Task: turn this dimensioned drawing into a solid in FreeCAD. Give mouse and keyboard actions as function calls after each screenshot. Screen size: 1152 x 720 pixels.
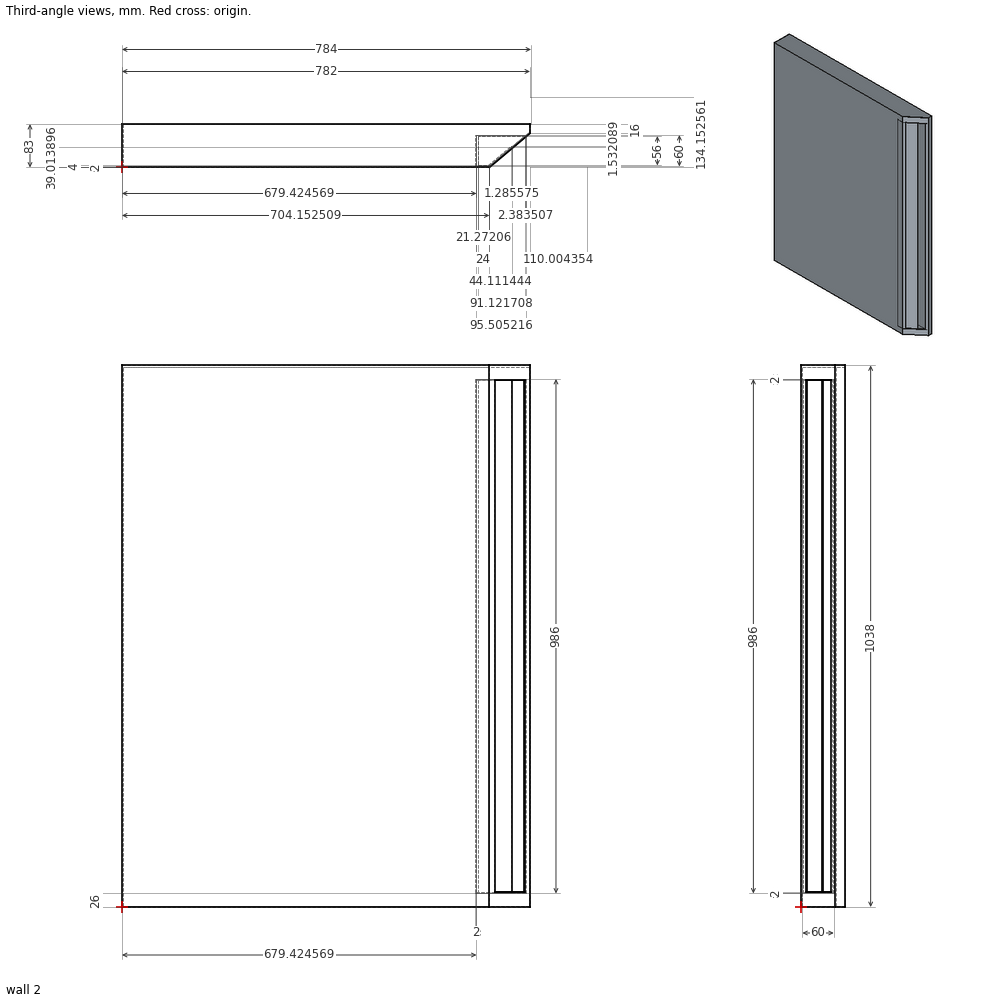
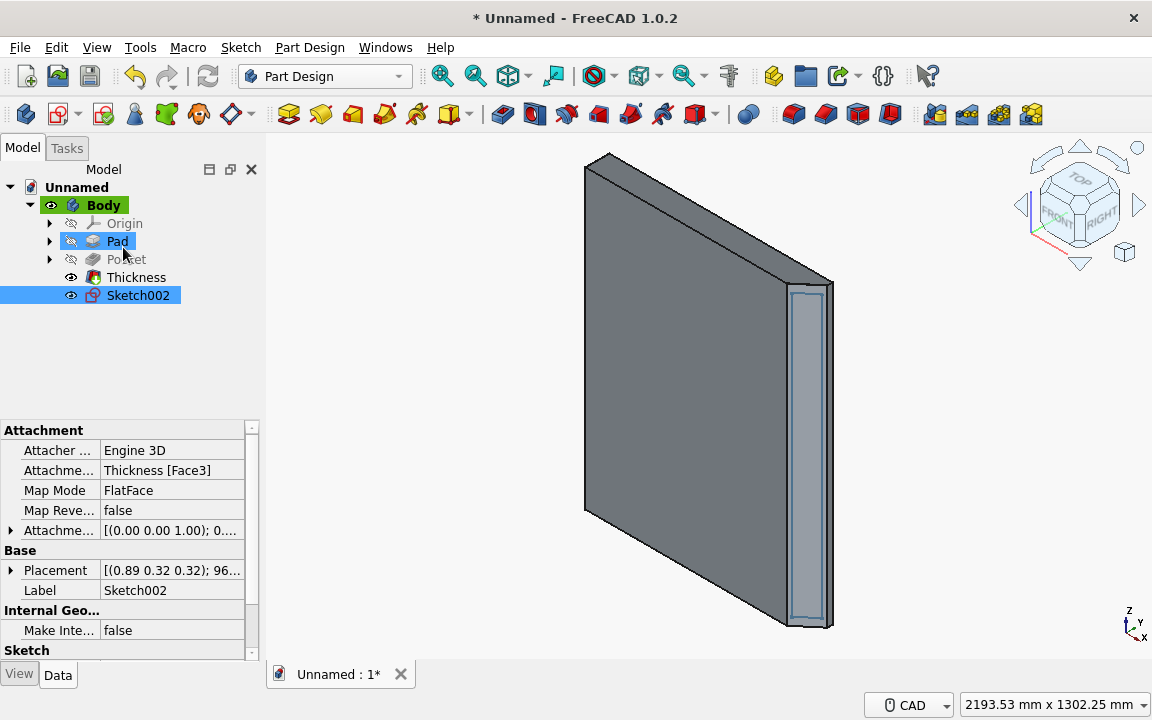
click(504, 114)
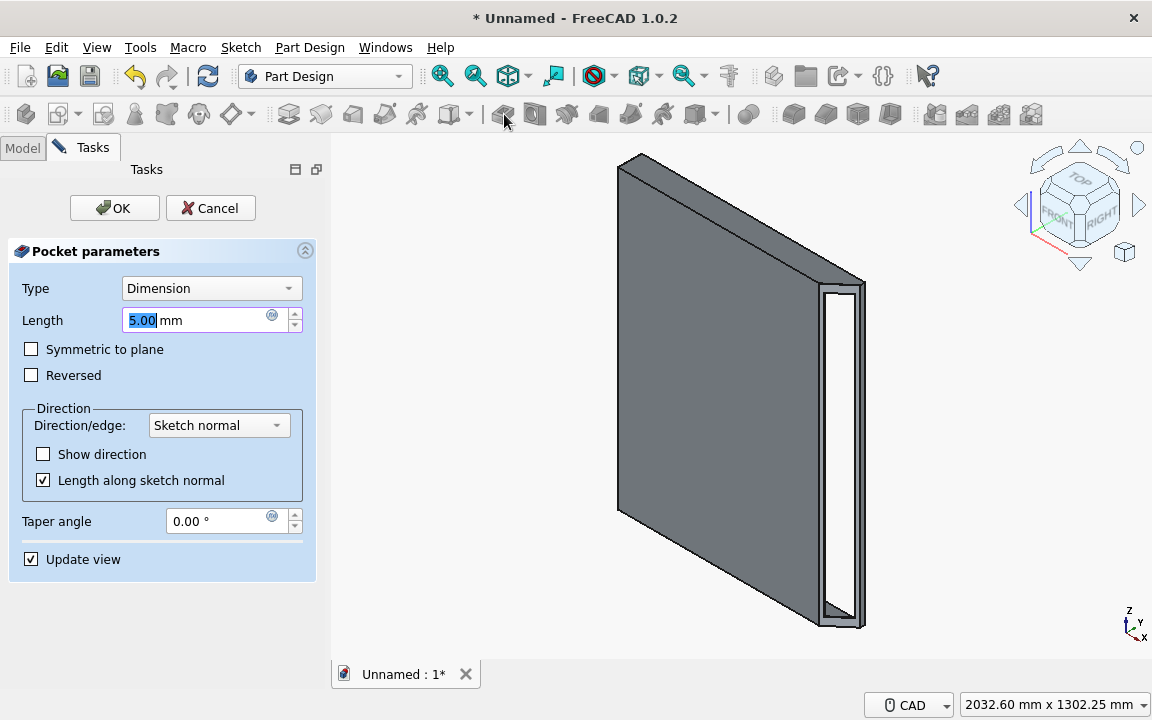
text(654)
key(Tab)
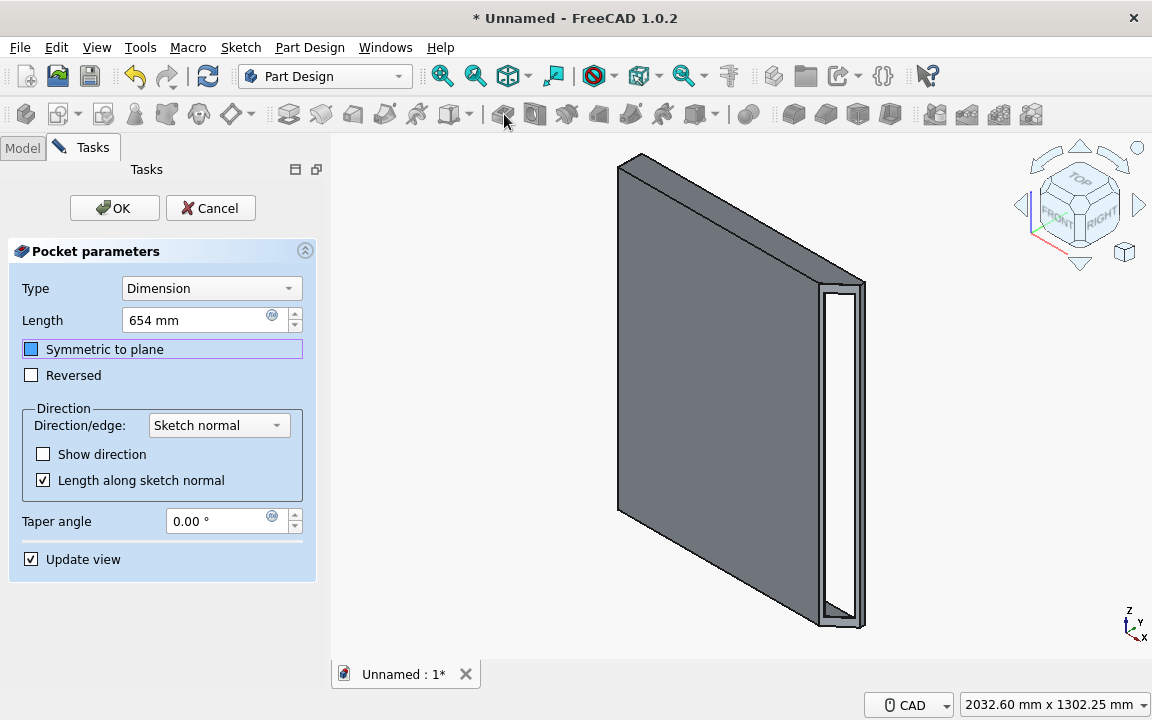
click(115, 208)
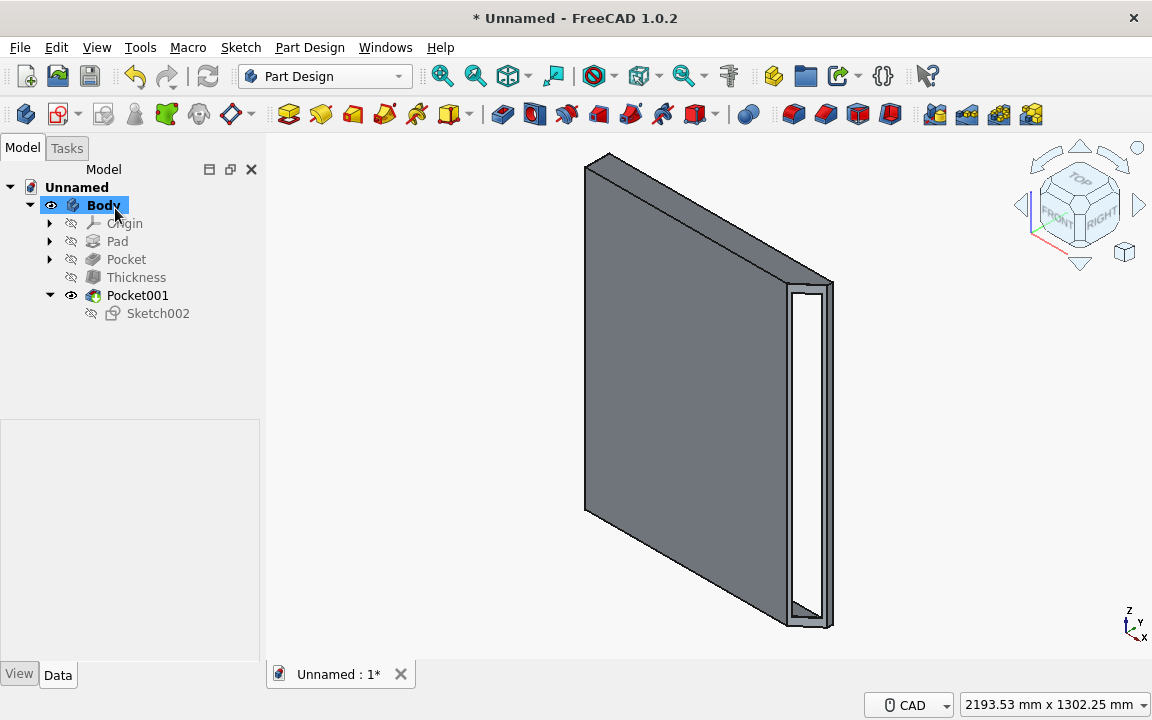
key(4)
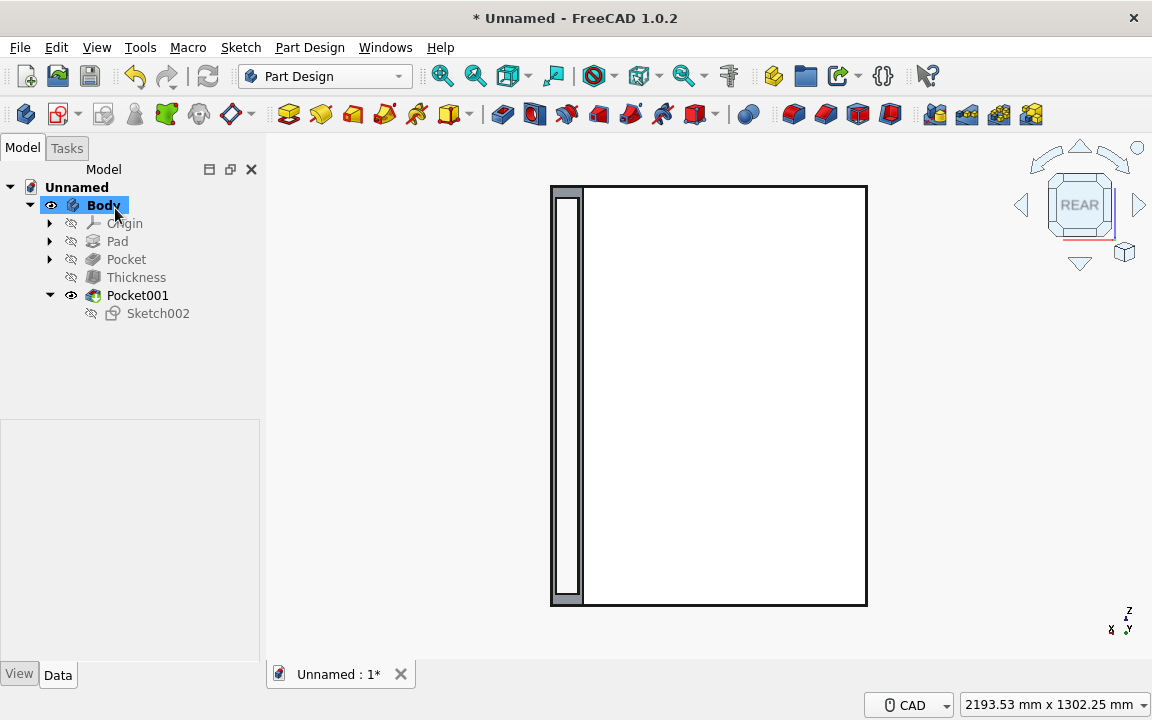
click(724, 335)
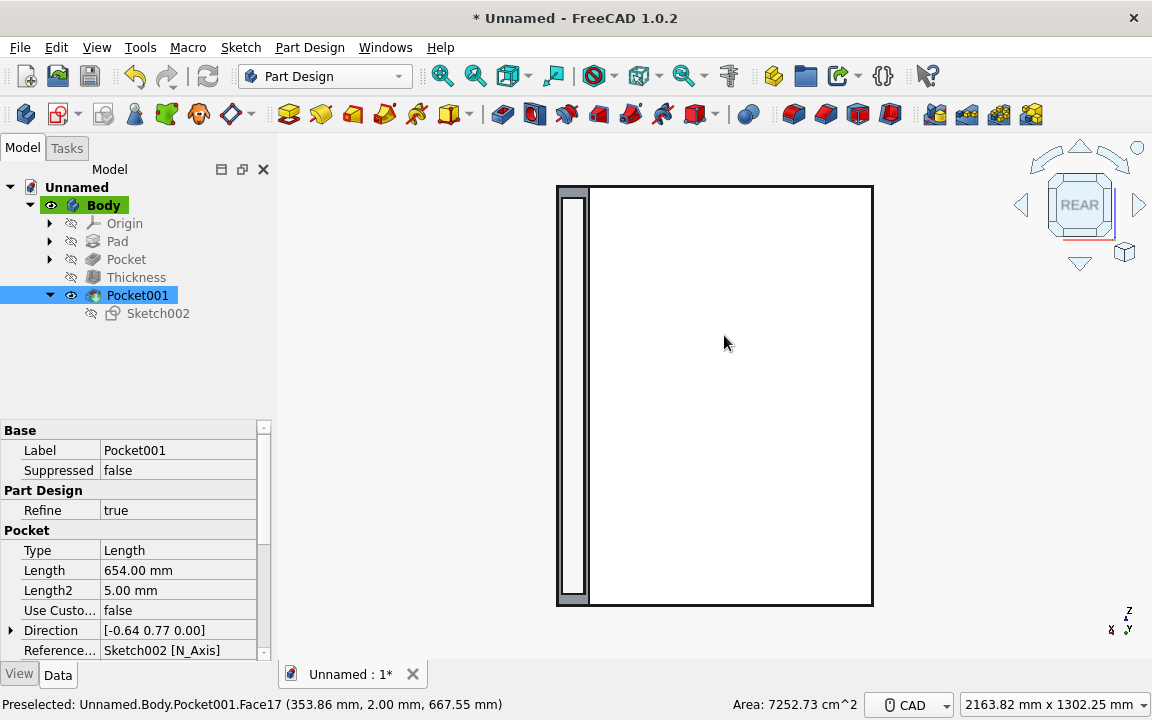
click(58, 114)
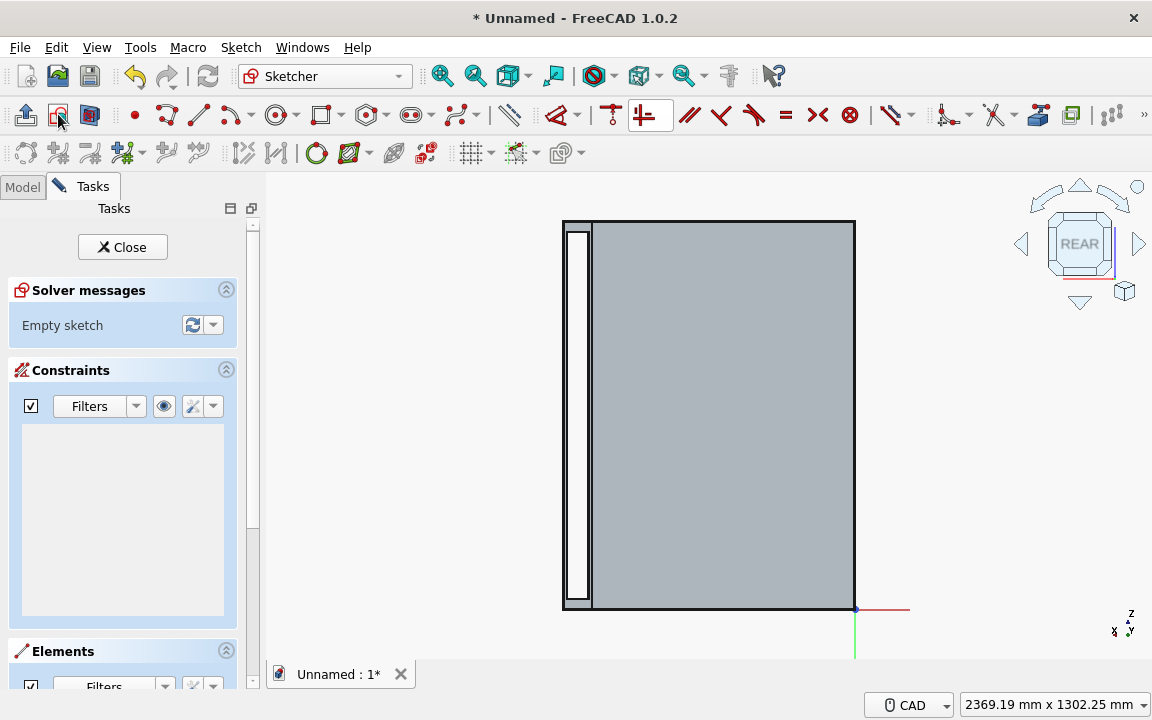
scroll(294, 394, down, 1)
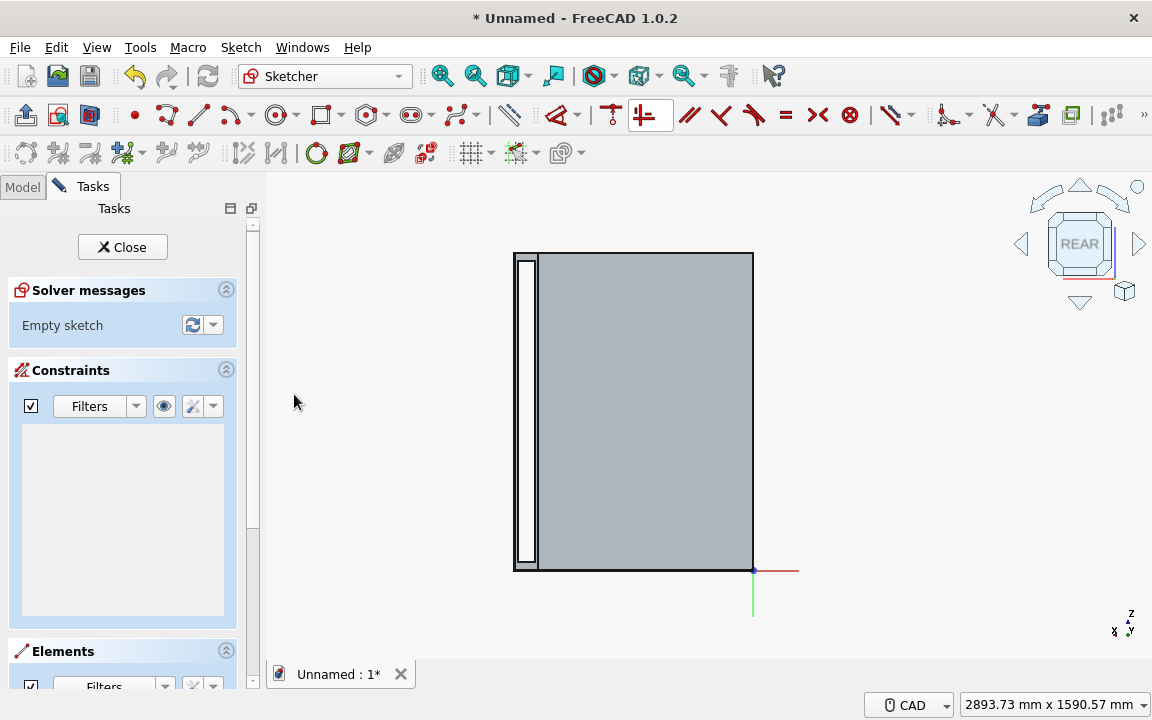
click(322, 116)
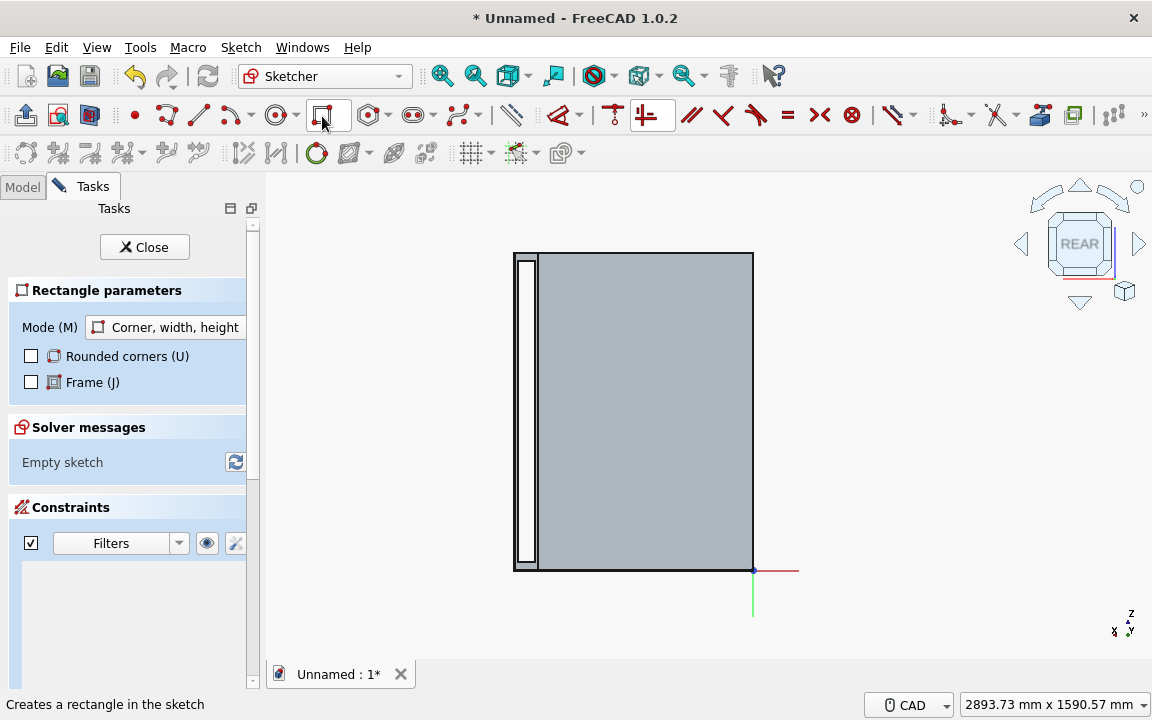
scroll(545, 261, up, 17)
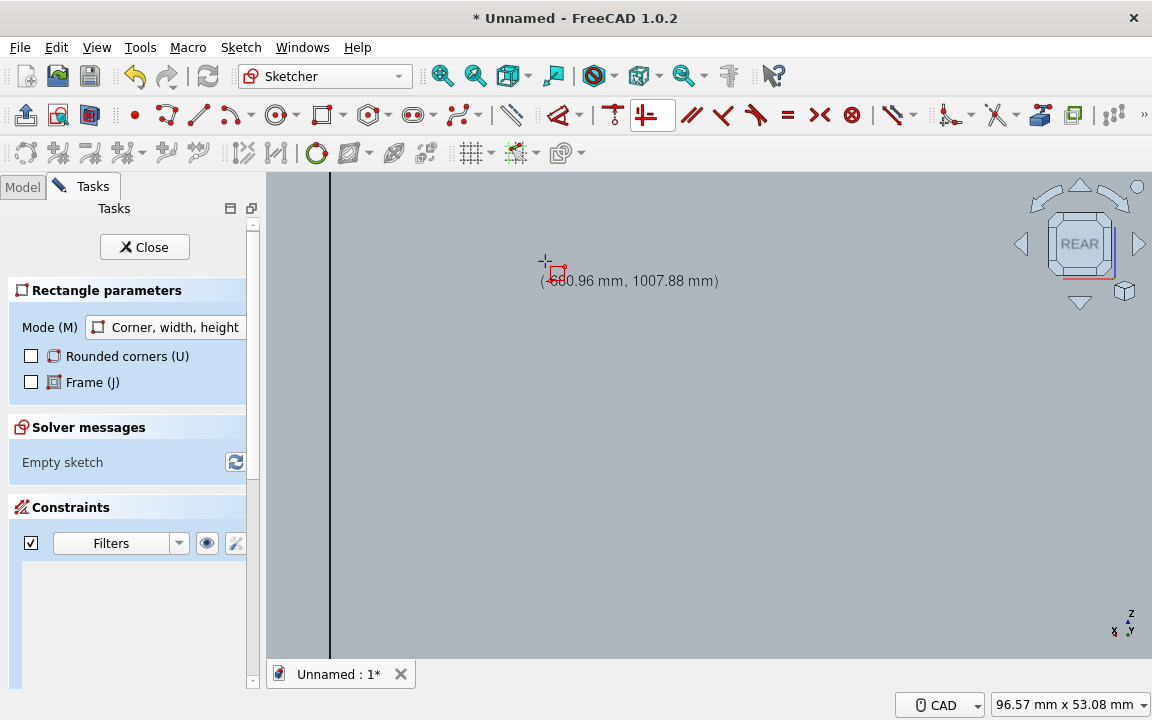
scroll(512, 225, down, 16)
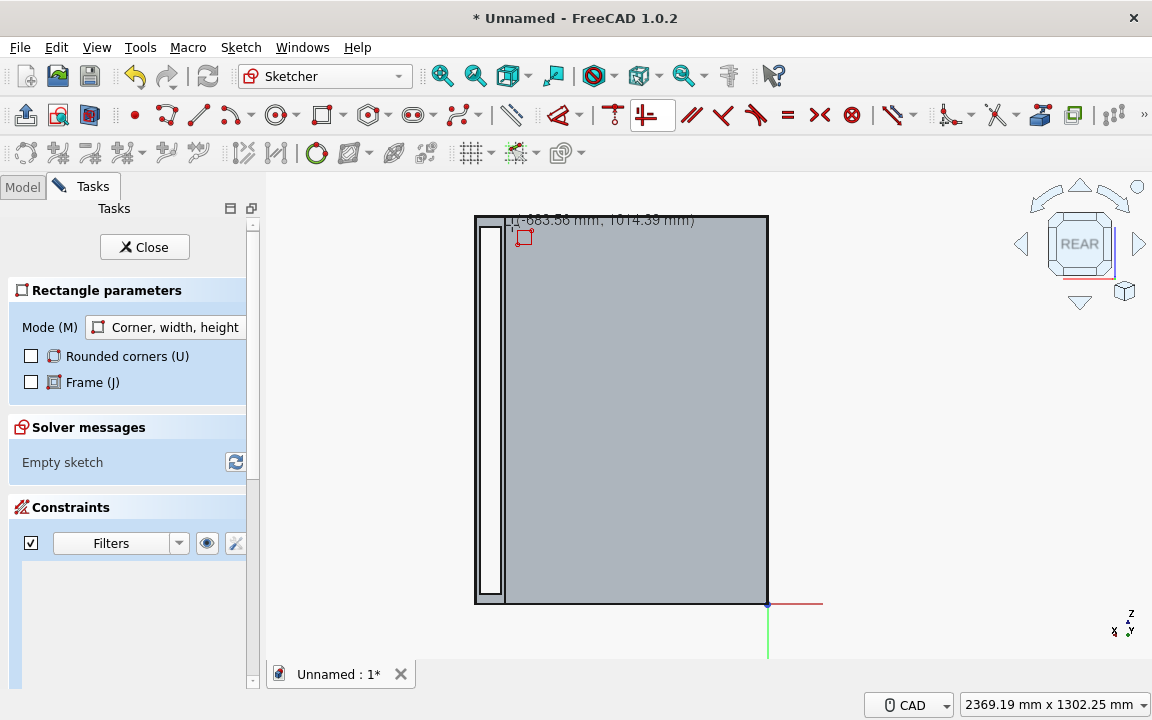
click(514, 226)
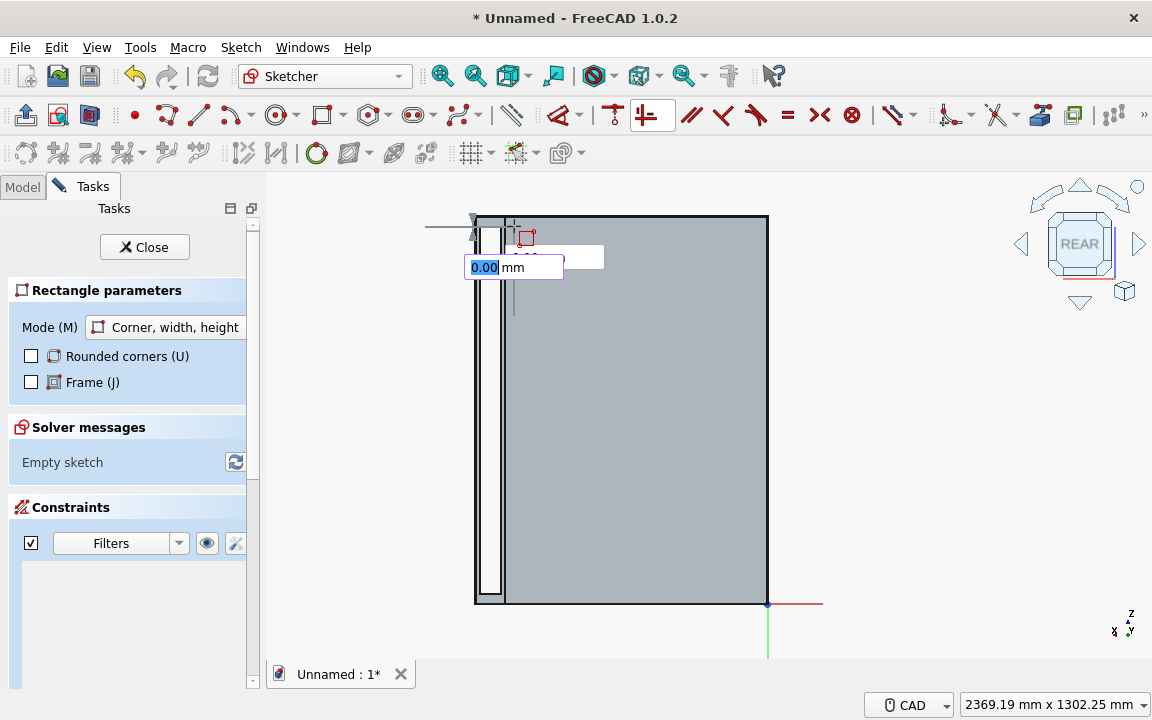
scroll(515, 595, up, 3)